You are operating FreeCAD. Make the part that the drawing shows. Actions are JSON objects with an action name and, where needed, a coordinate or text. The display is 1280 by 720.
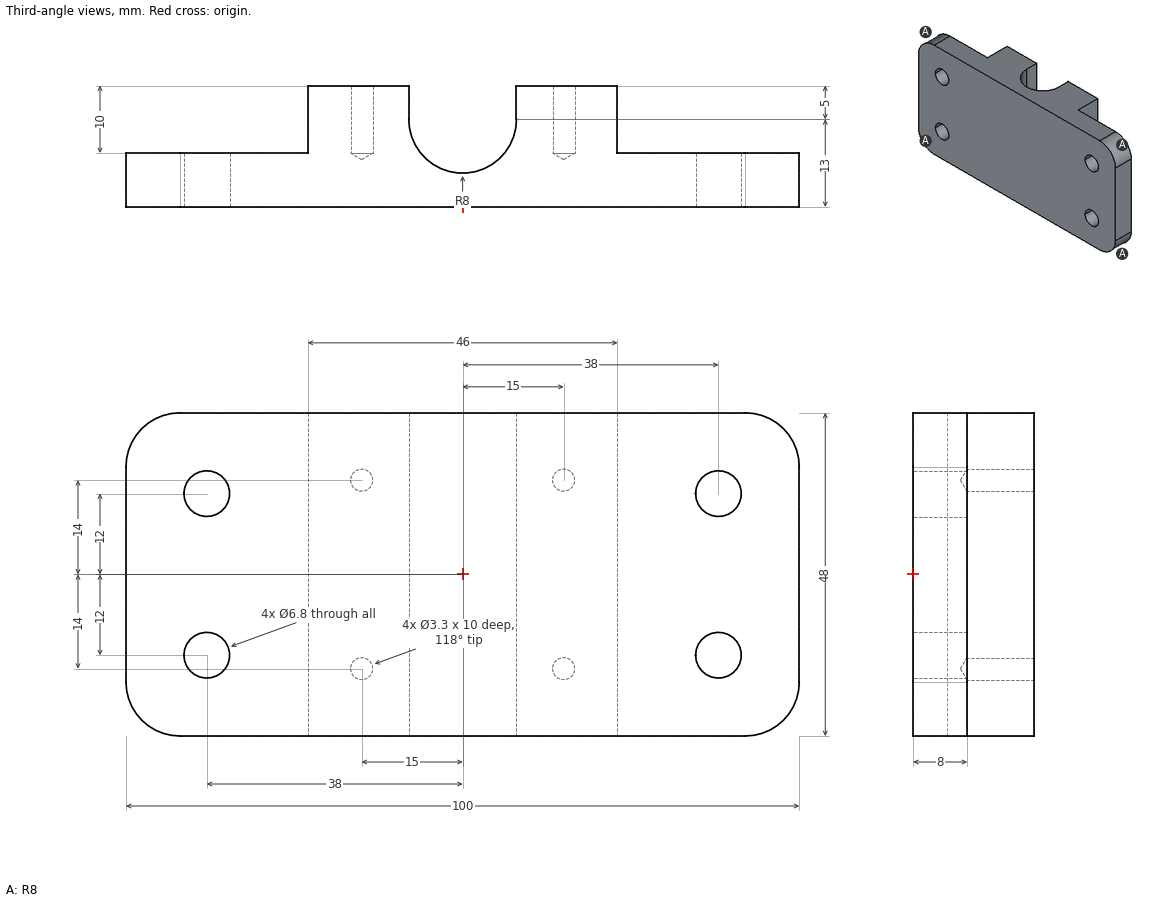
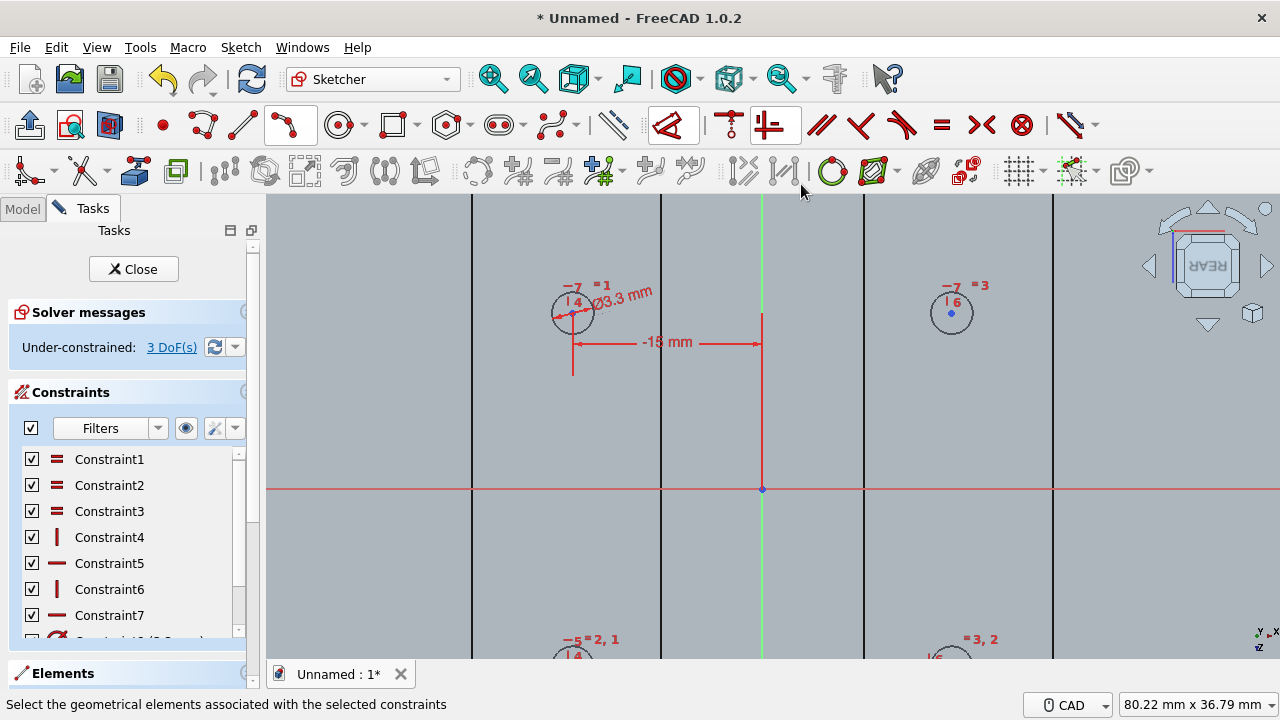
{"action": "left_click", "coordinate": [573, 313]}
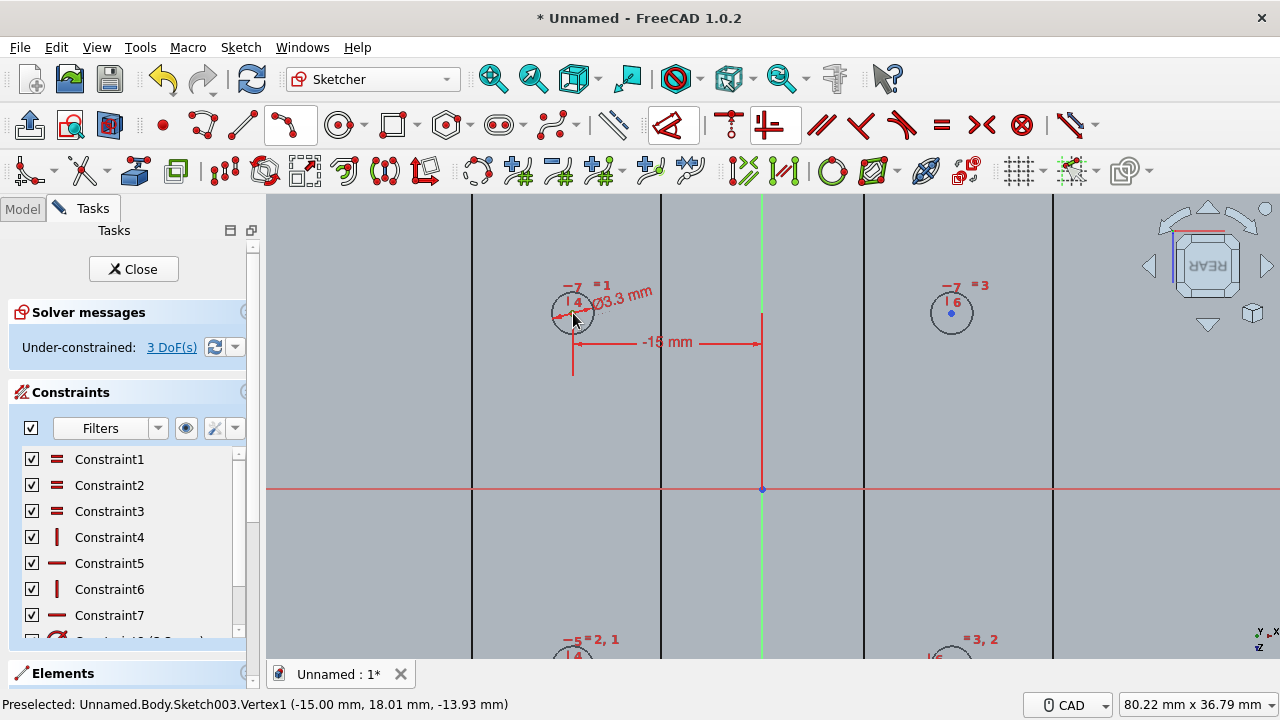
{"action": "key", "text": "i"}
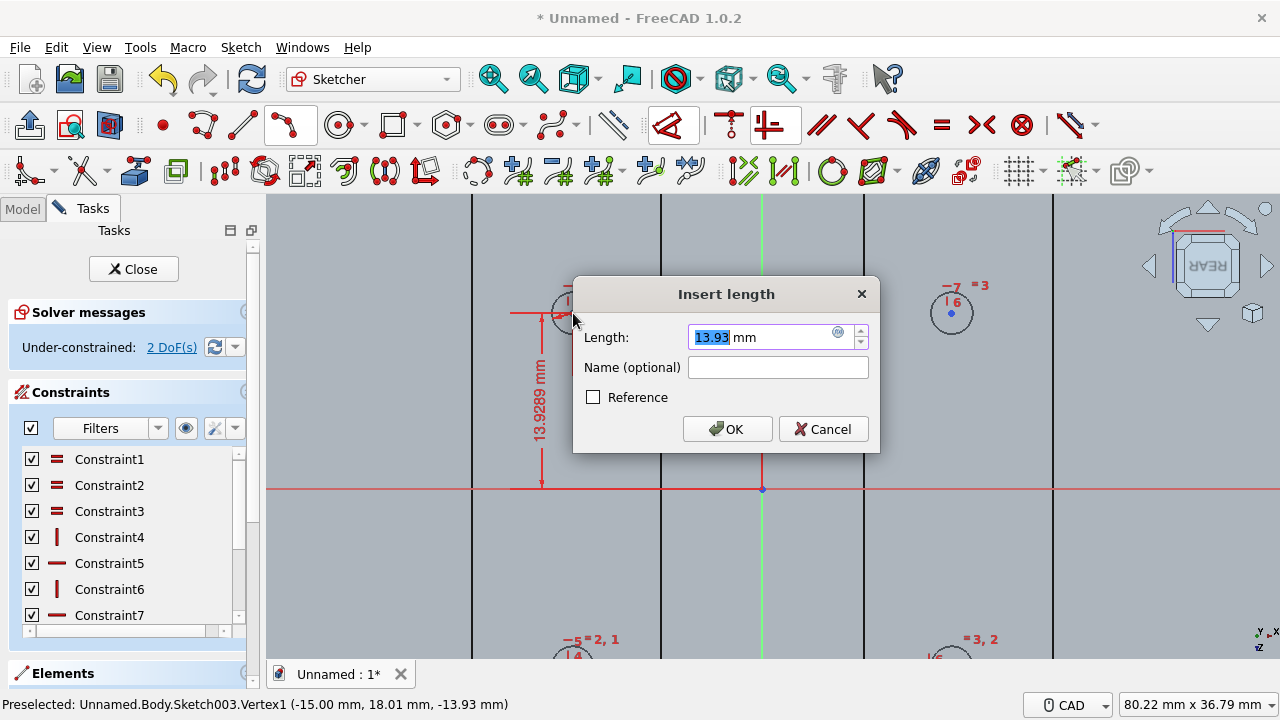
{"action": "type", "text": "14"}
{"action": "key", "text": "Return"}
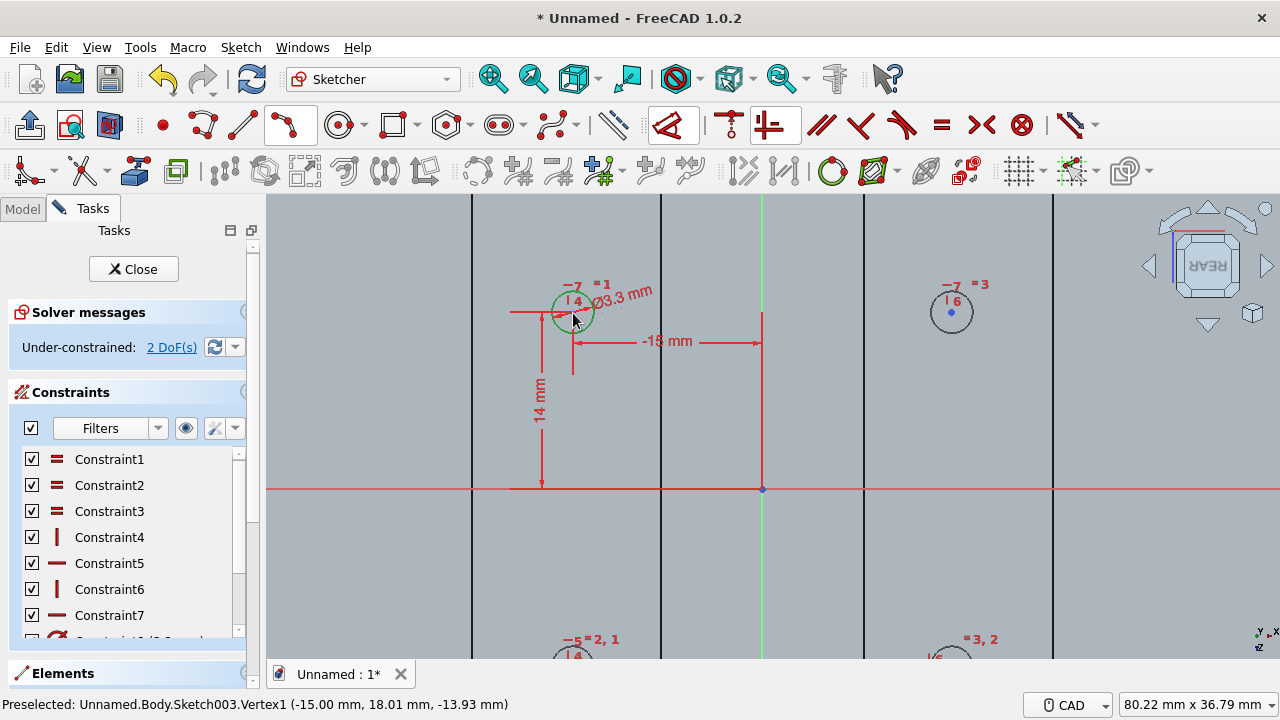
{"action": "scroll", "coordinate": [587, 299], "scroll_direction": "down", "scroll_amount": 2}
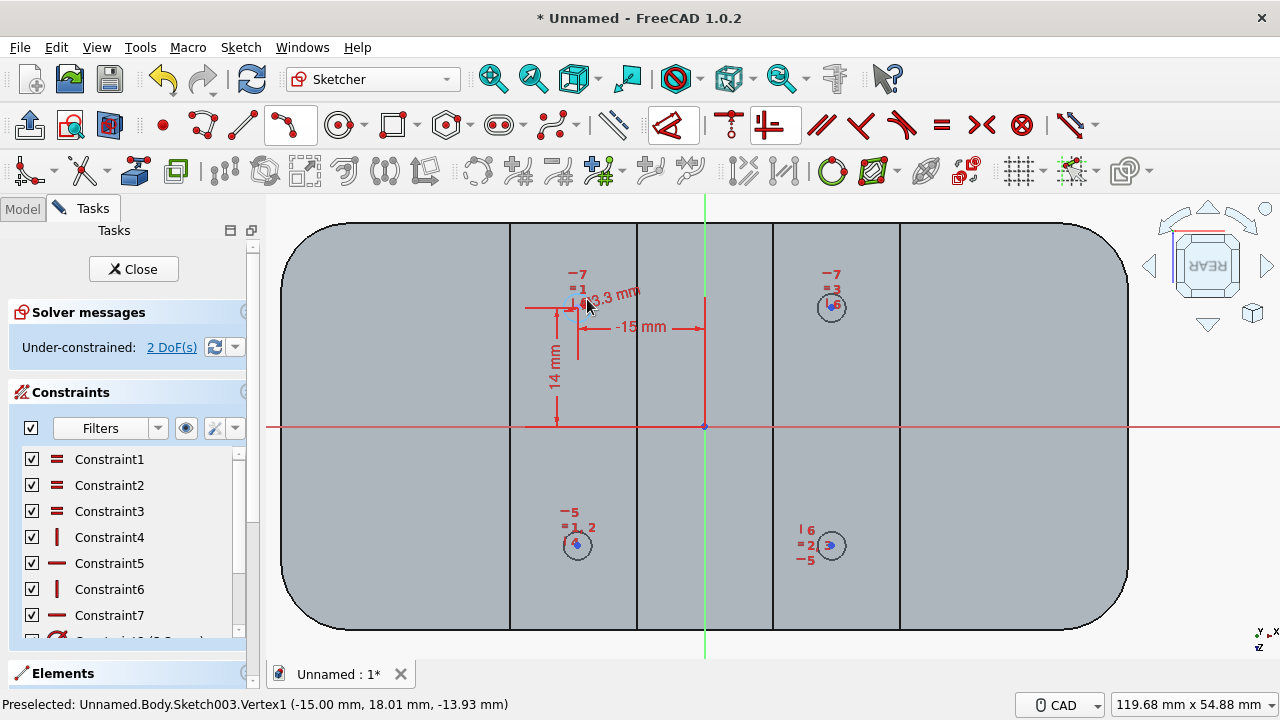
{"action": "left_click", "coordinate": [578, 546]}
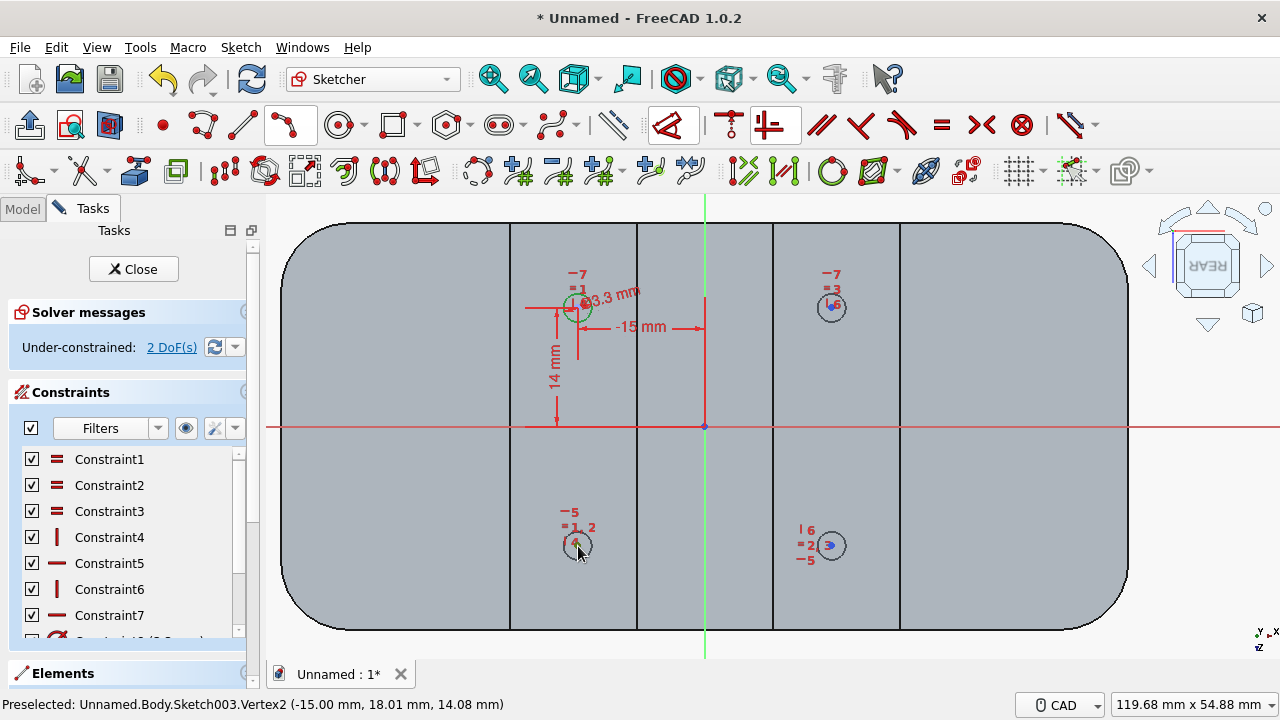
{"action": "key", "text": "i"}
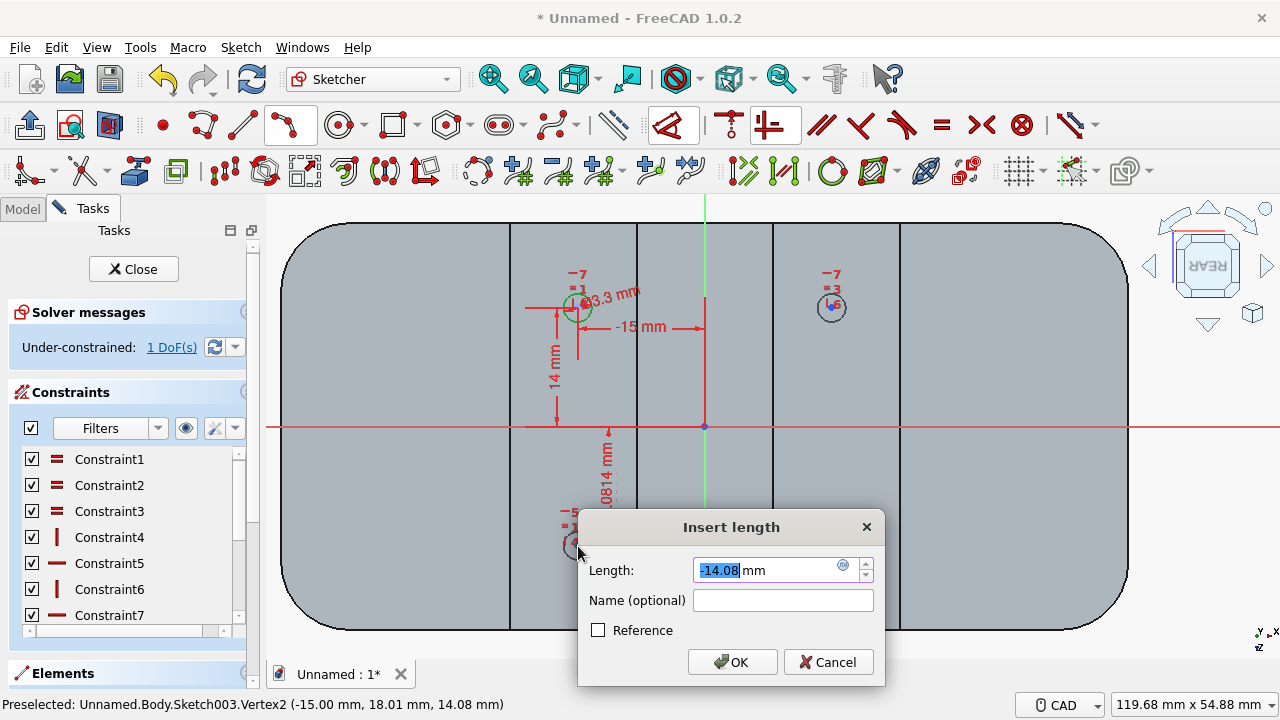
{"action": "type", "text": "-14"}
{"action": "key", "text": "Return"}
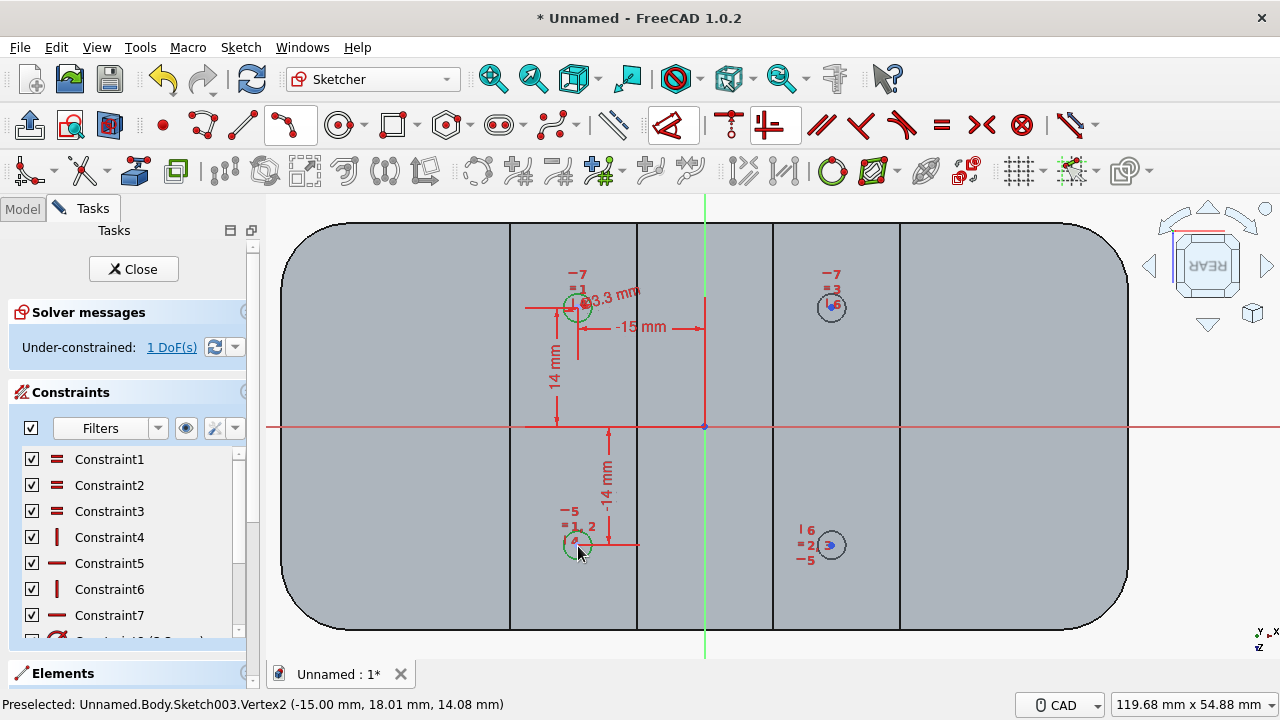
{"action": "left_click", "coordinate": [832, 545]}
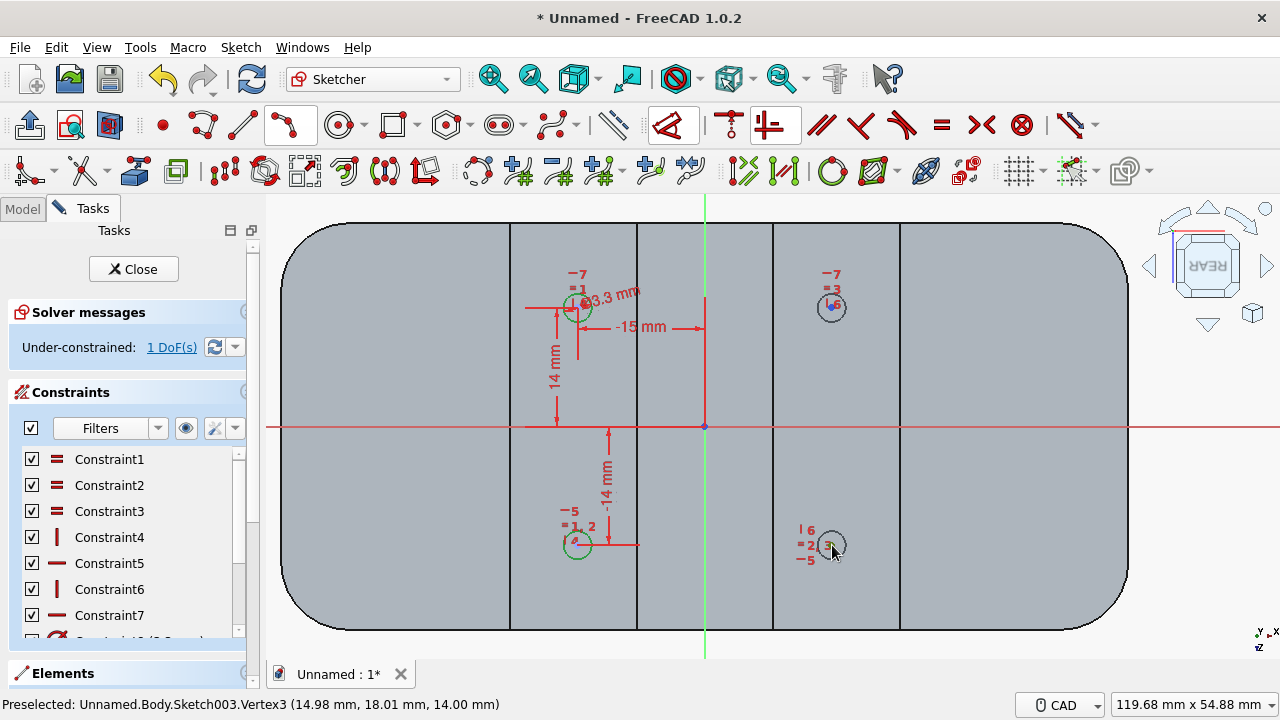
{"action": "key", "text": "l"}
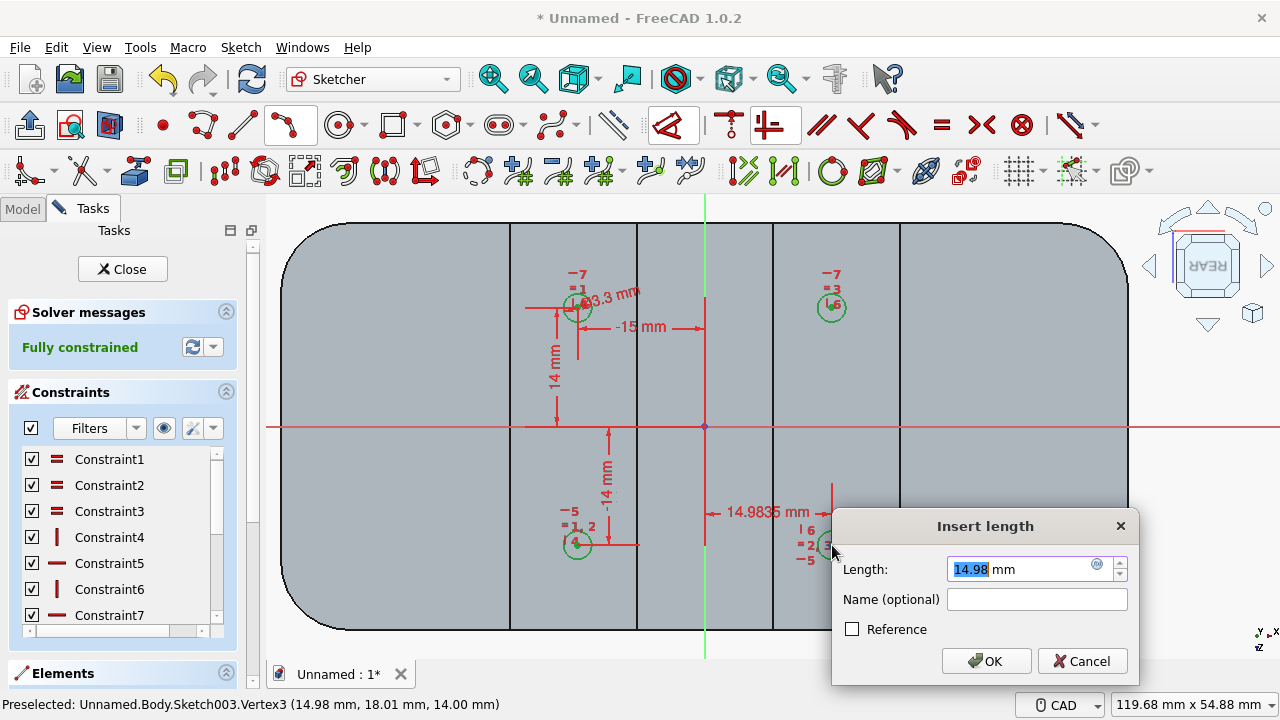
{"action": "type", "text": "15"}
{"action": "key", "text": "Return"}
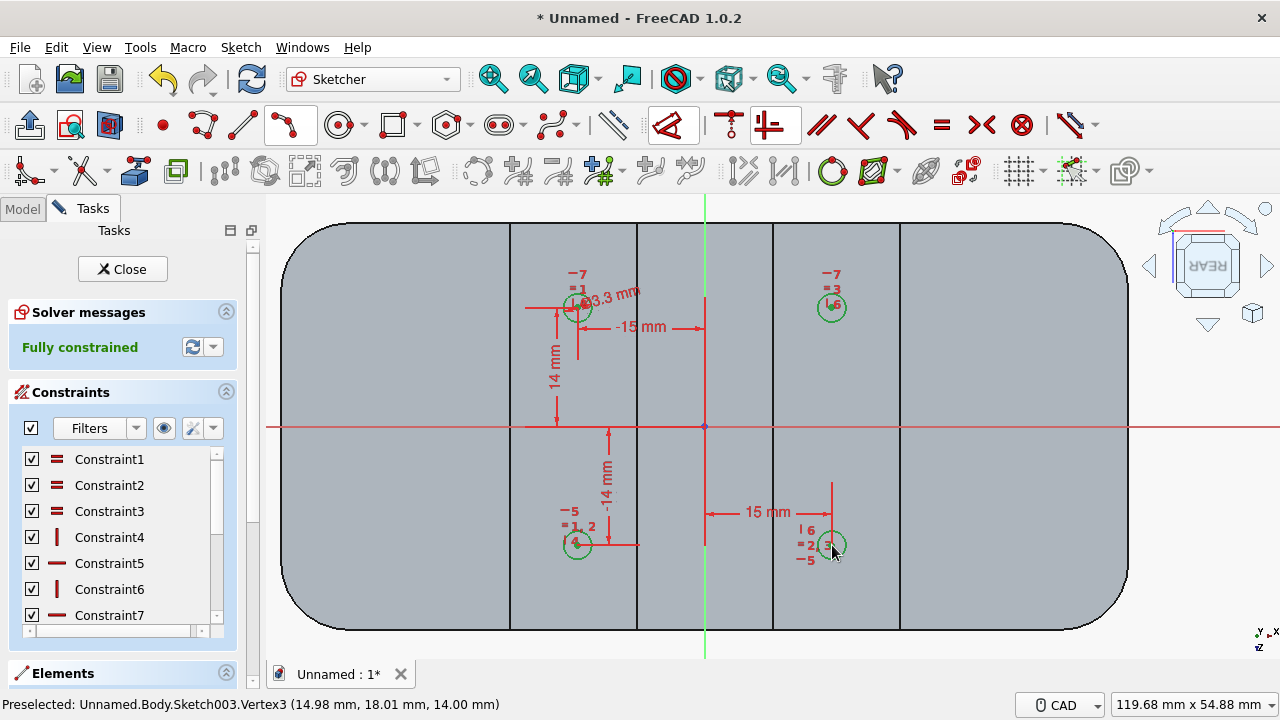
{"action": "left_click", "coordinate": [123, 269]}